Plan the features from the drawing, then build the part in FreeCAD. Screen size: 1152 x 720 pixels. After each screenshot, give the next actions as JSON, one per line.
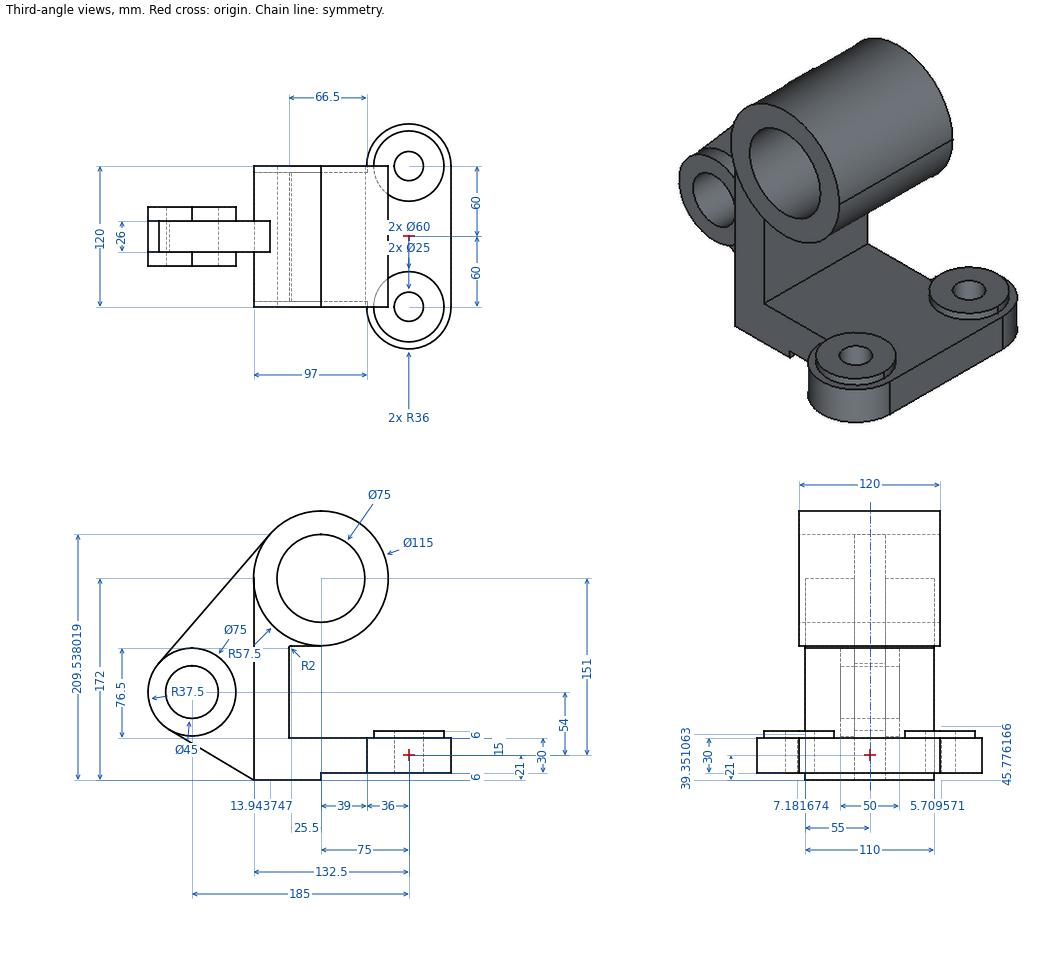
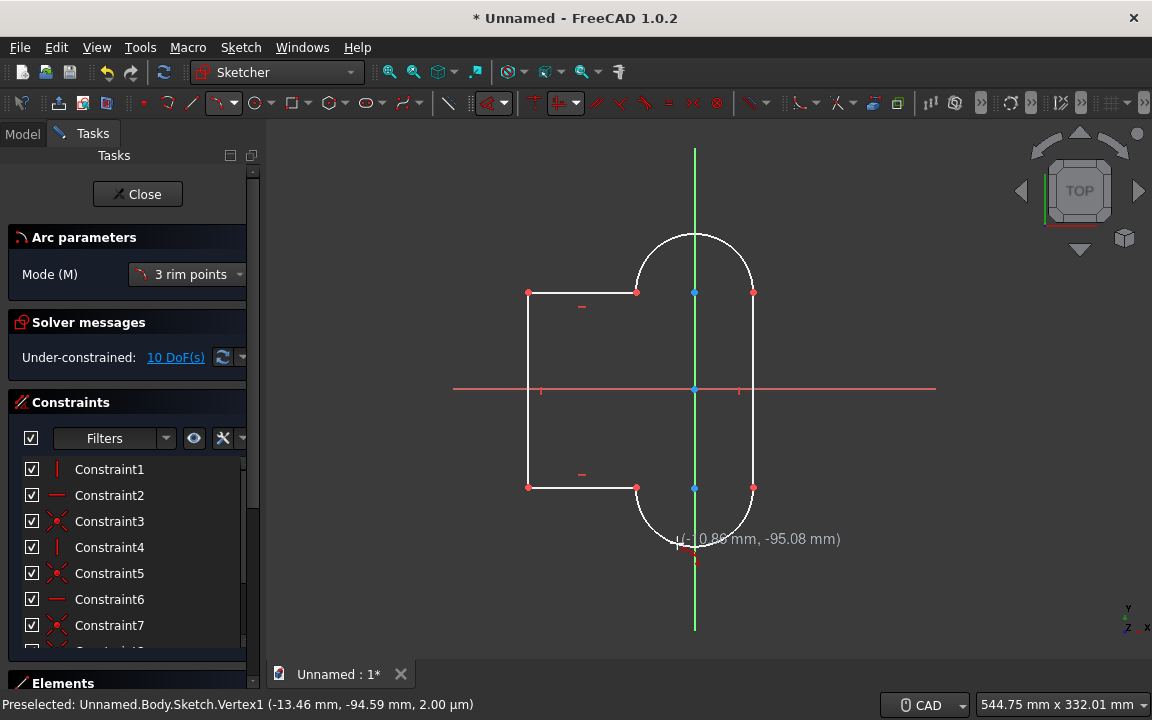
{"action": "left_click", "coordinate": [256, 104]}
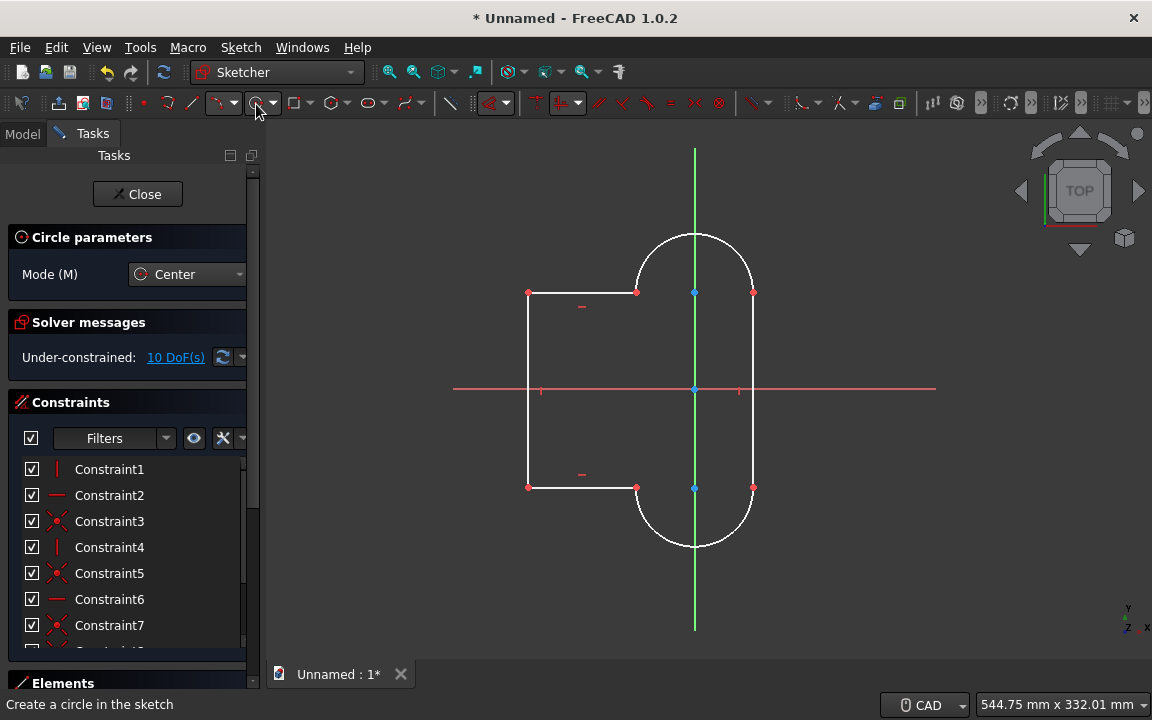
{"action": "left_click", "coordinate": [695, 487]}
{"action": "left_click", "coordinate": [709, 473]}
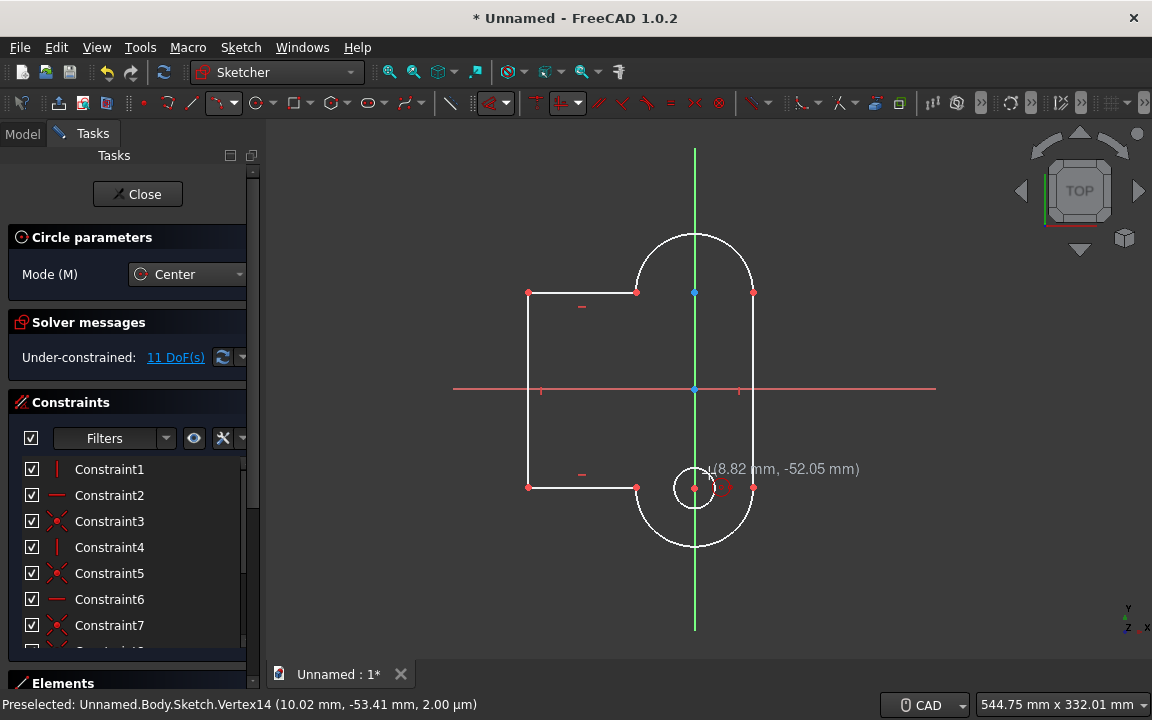
{"action": "left_click", "coordinate": [695, 292]}
{"action": "left_click", "coordinate": [709, 277]}
{"action": "key", "text": "Escape"}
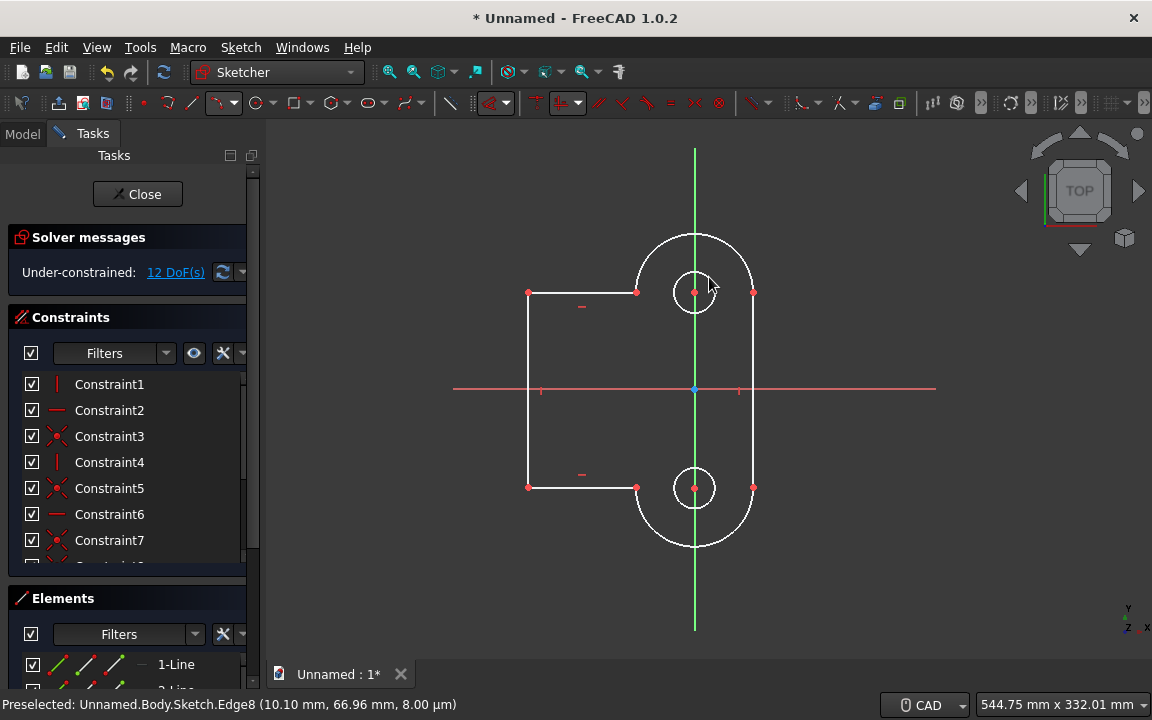
{"action": "left_click", "coordinate": [753, 429]}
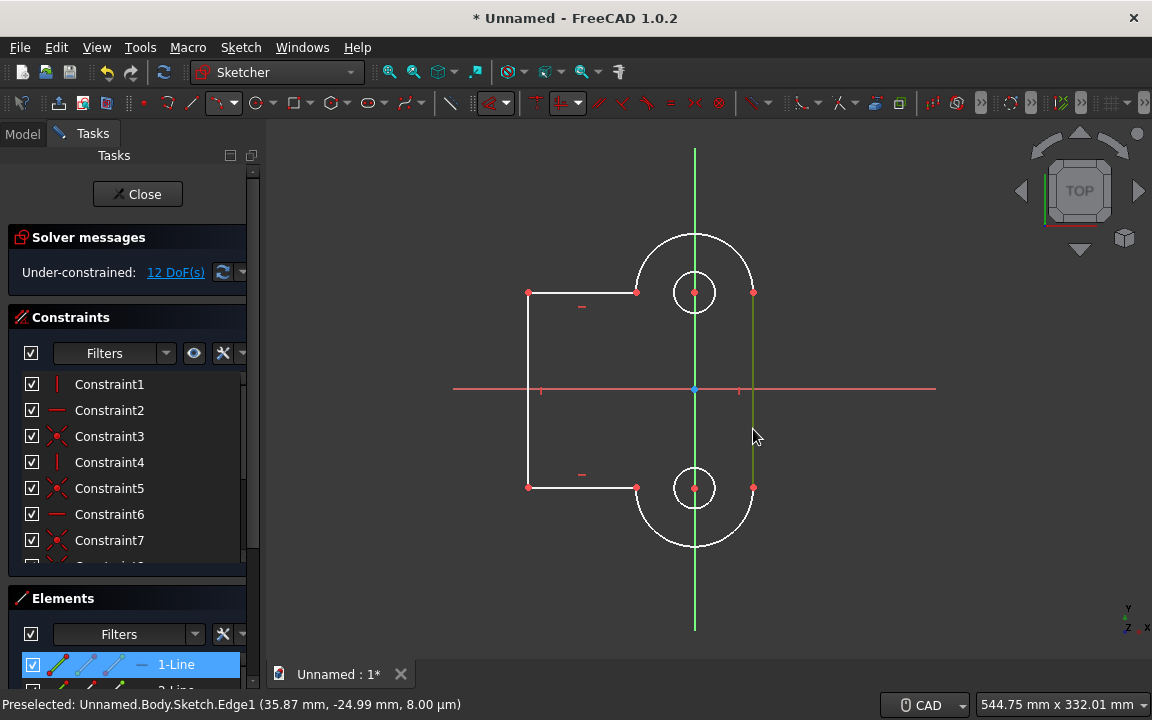
{"action": "left_click", "coordinate": [729, 245]}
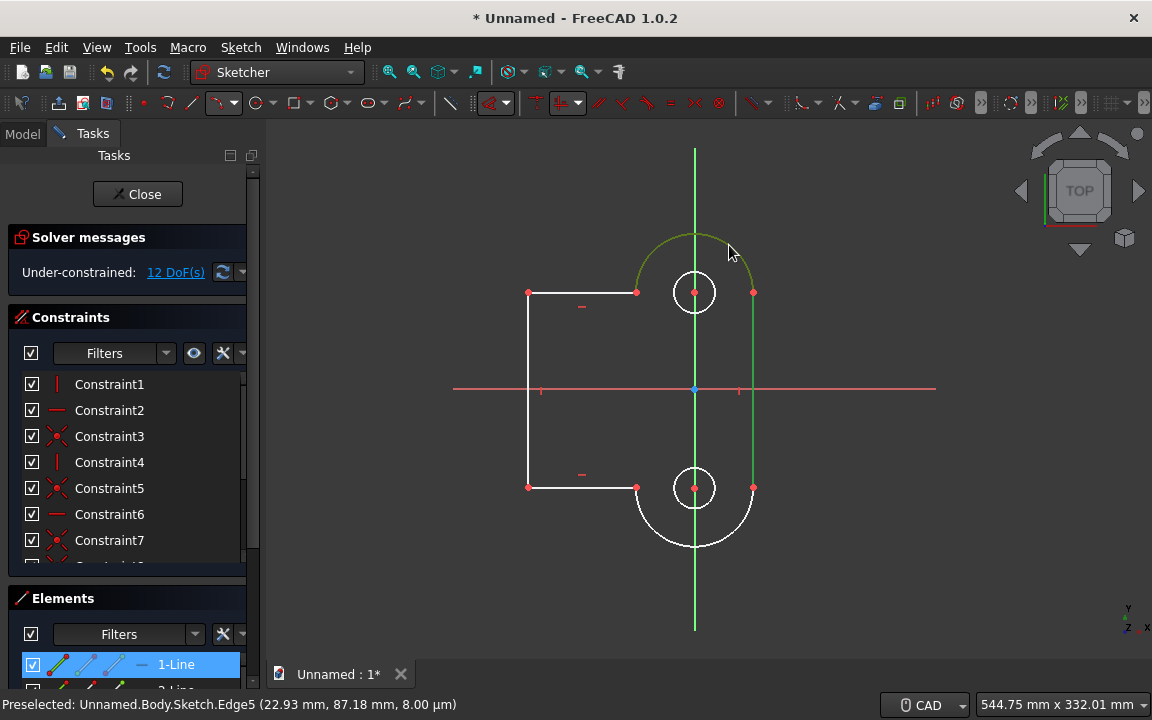
{"action": "key", "text": "t"}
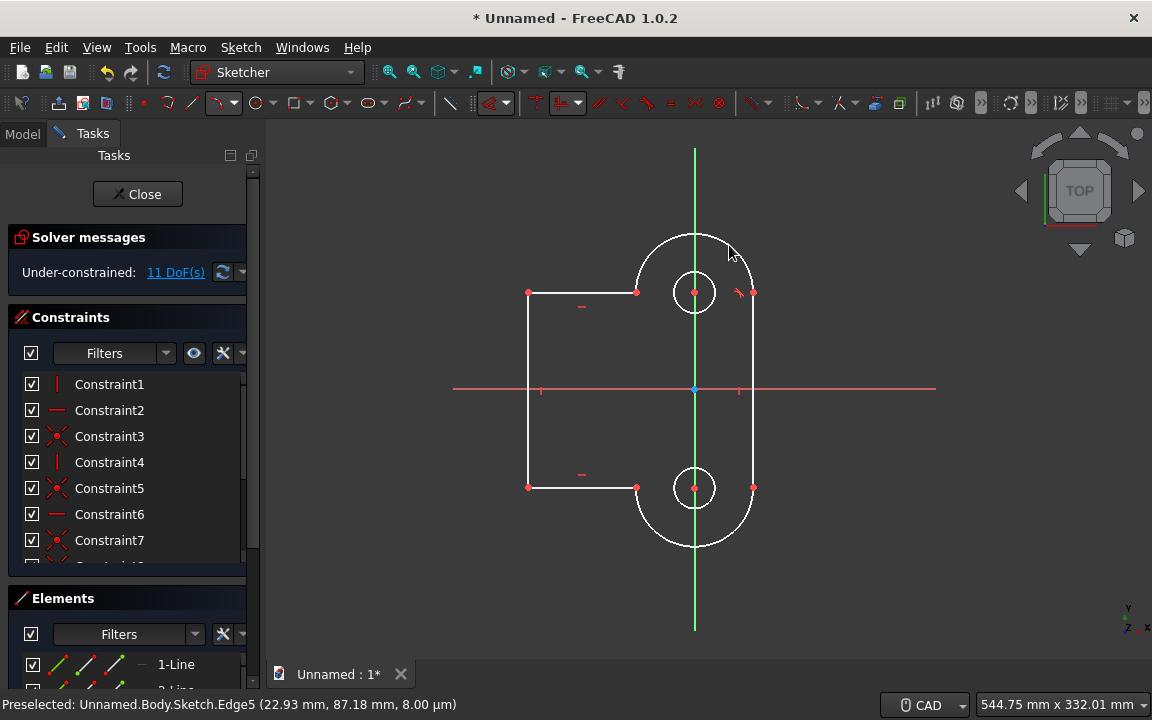
{"action": "left_click", "coordinate": [753, 429]}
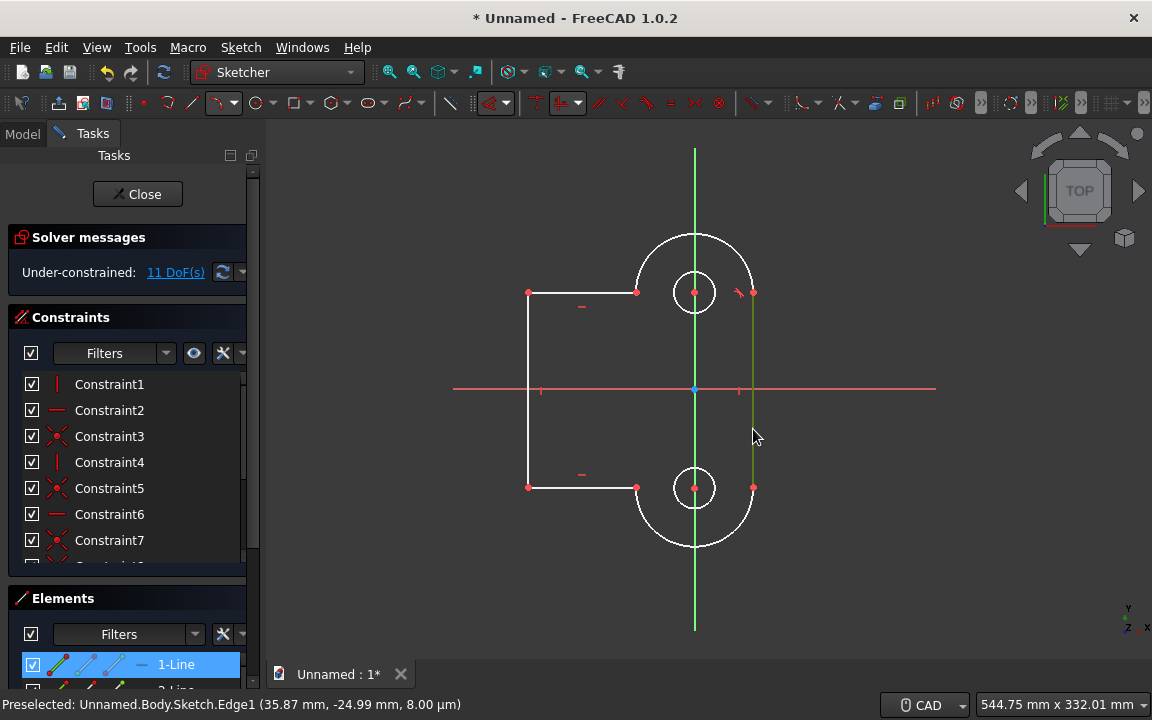
{"action": "left_click", "coordinate": [660, 535]}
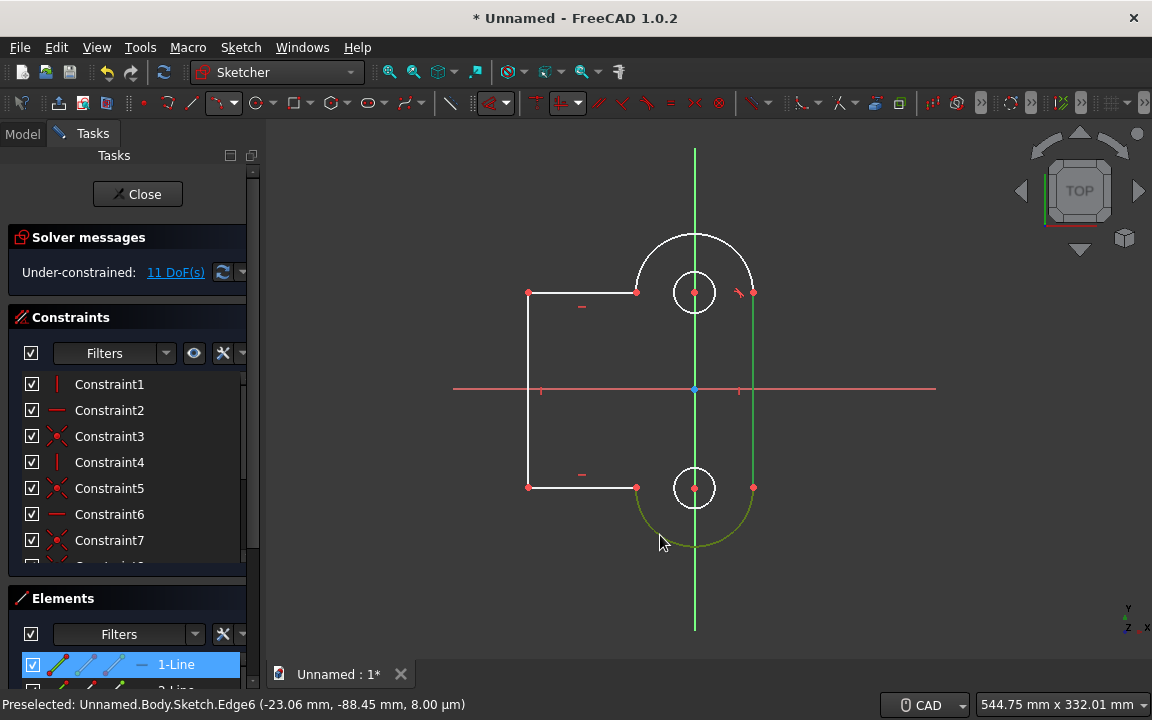
{"action": "key", "text": "t"}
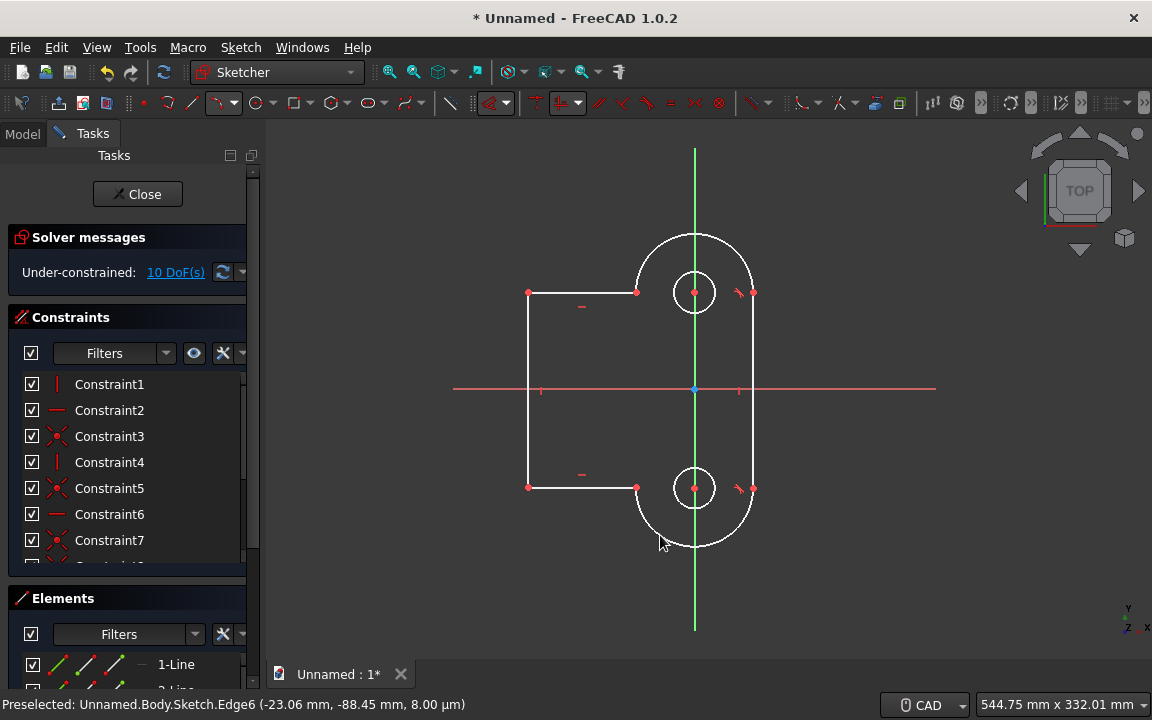
{"action": "left_click", "coordinate": [729, 245]}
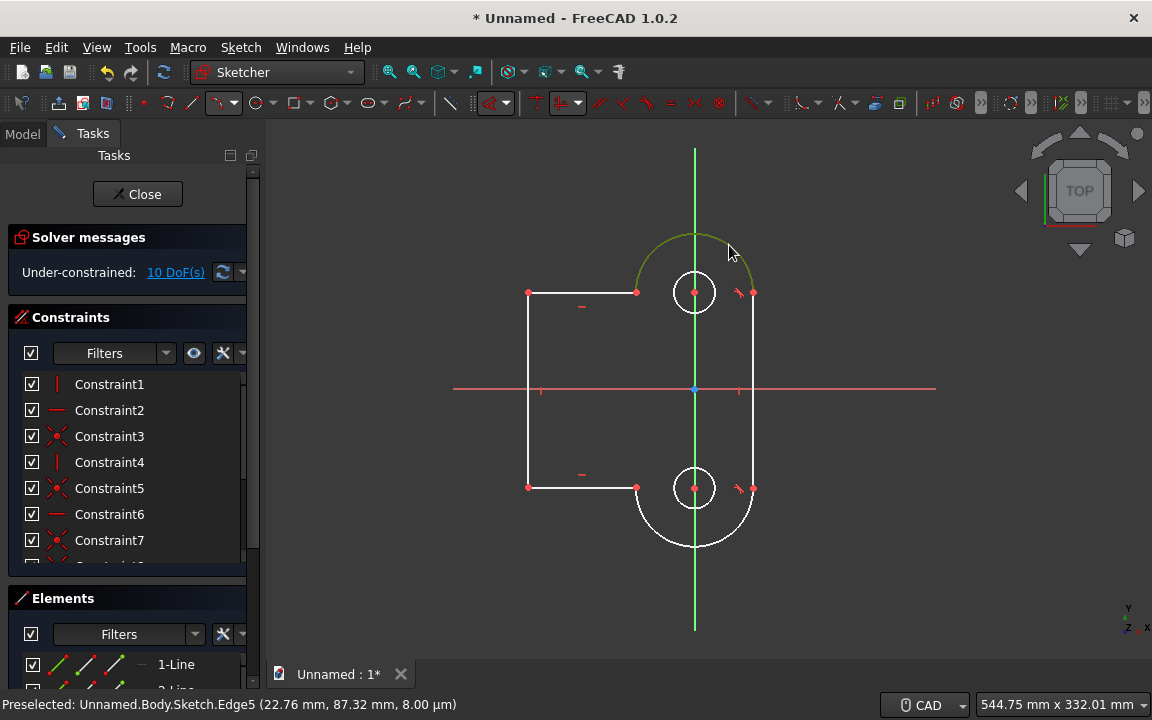
{"action": "left_click", "coordinate": [660, 535]}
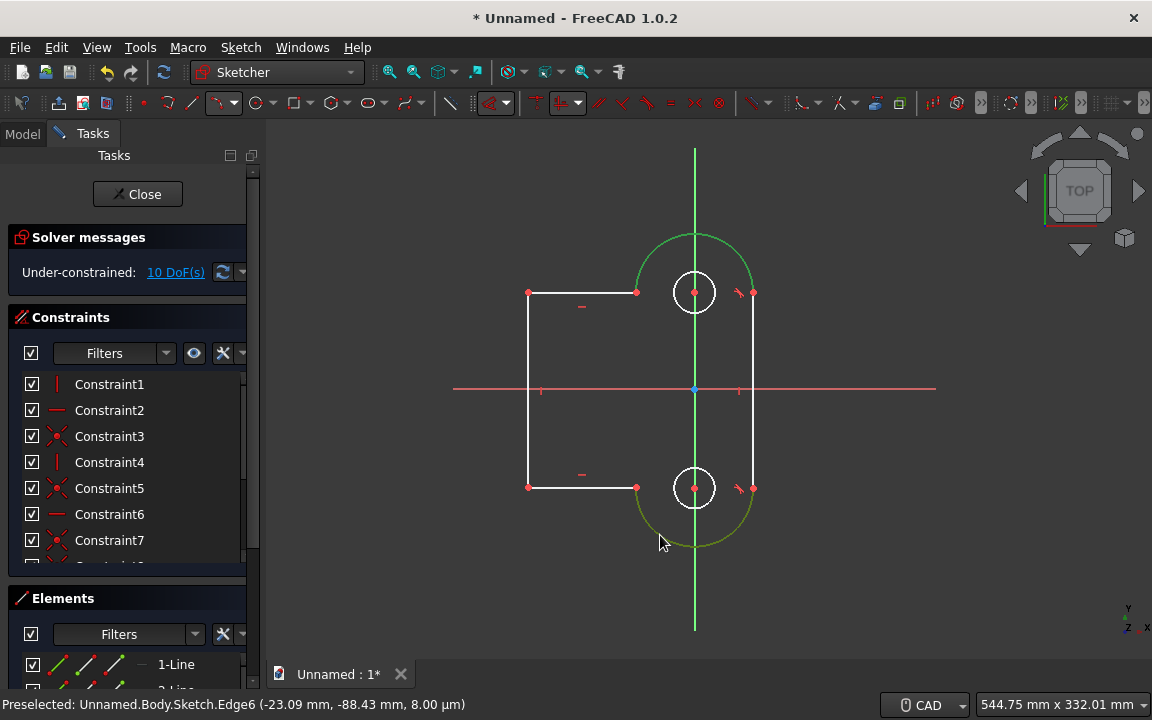
{"action": "left_click", "coordinate": [672, 104]}